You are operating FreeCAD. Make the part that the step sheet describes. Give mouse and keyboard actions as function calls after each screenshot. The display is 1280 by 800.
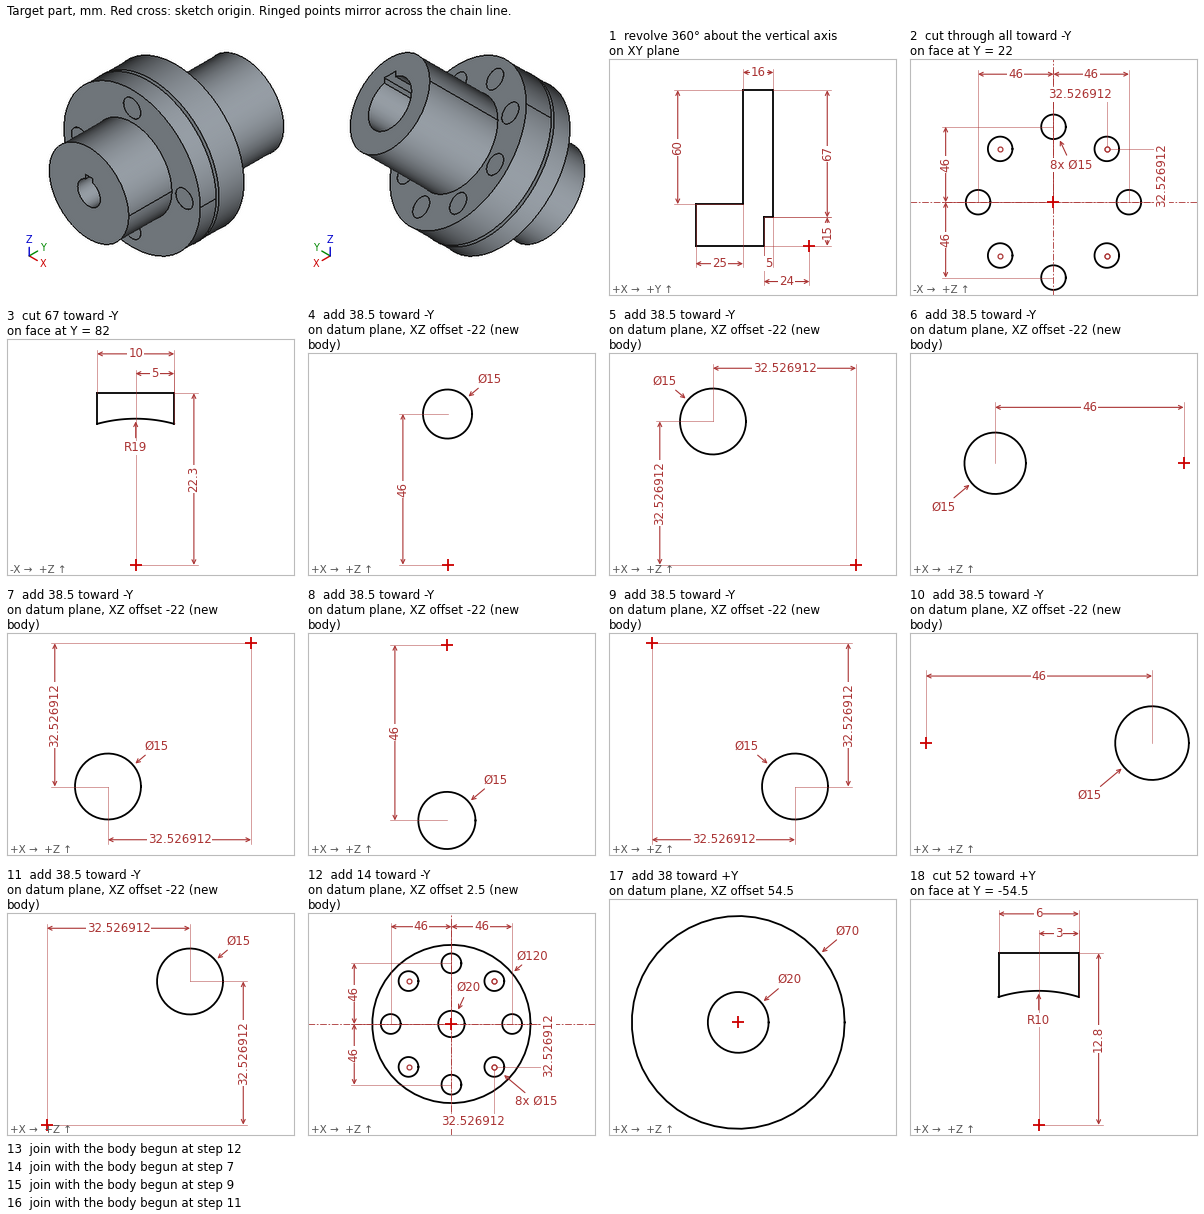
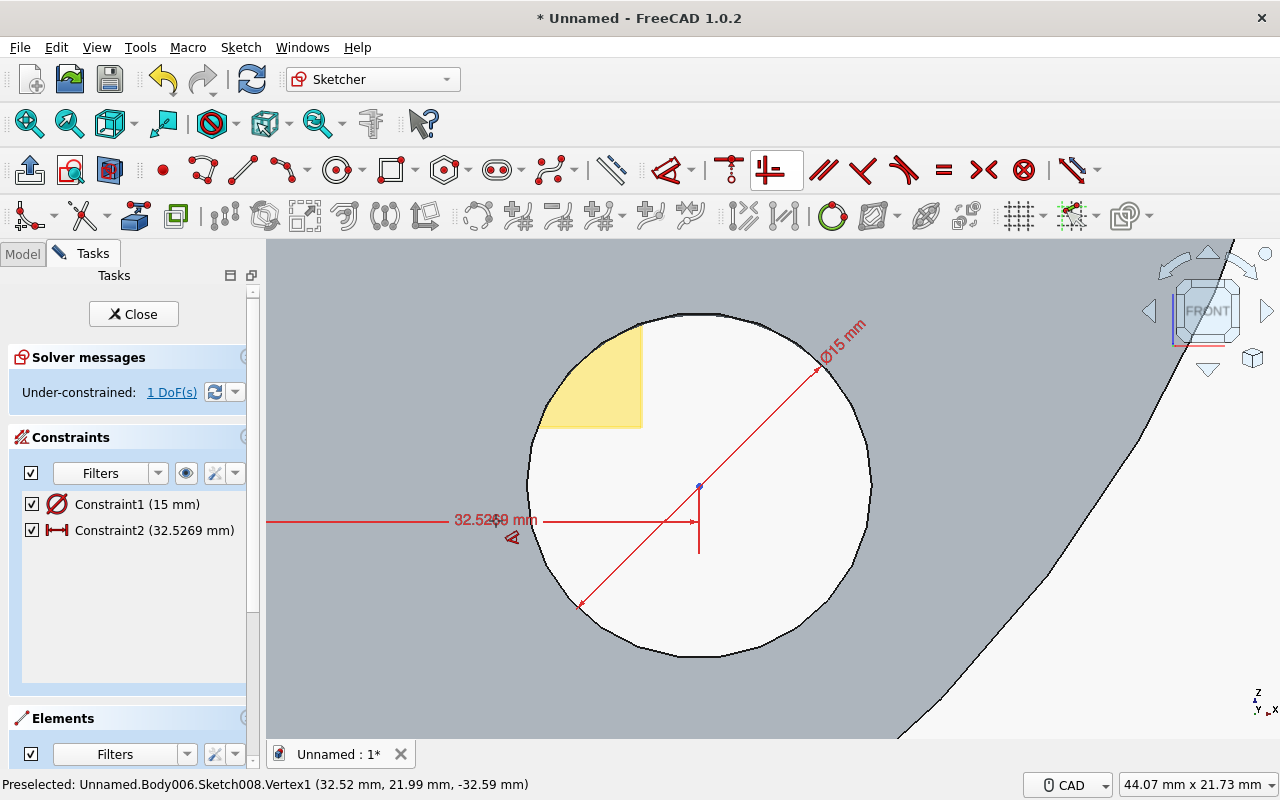
click(699, 487)
click(733, 377)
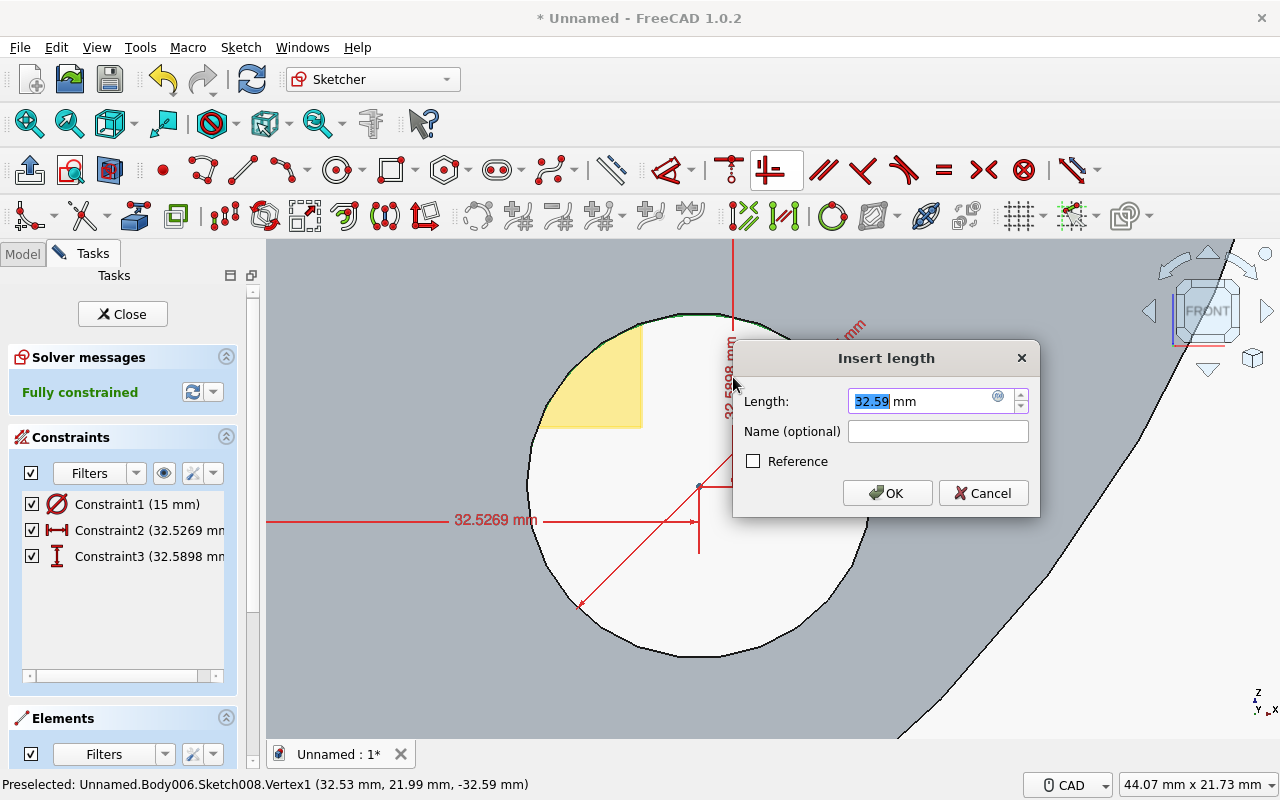
text(32.526912)
key(Return)
key(Escape)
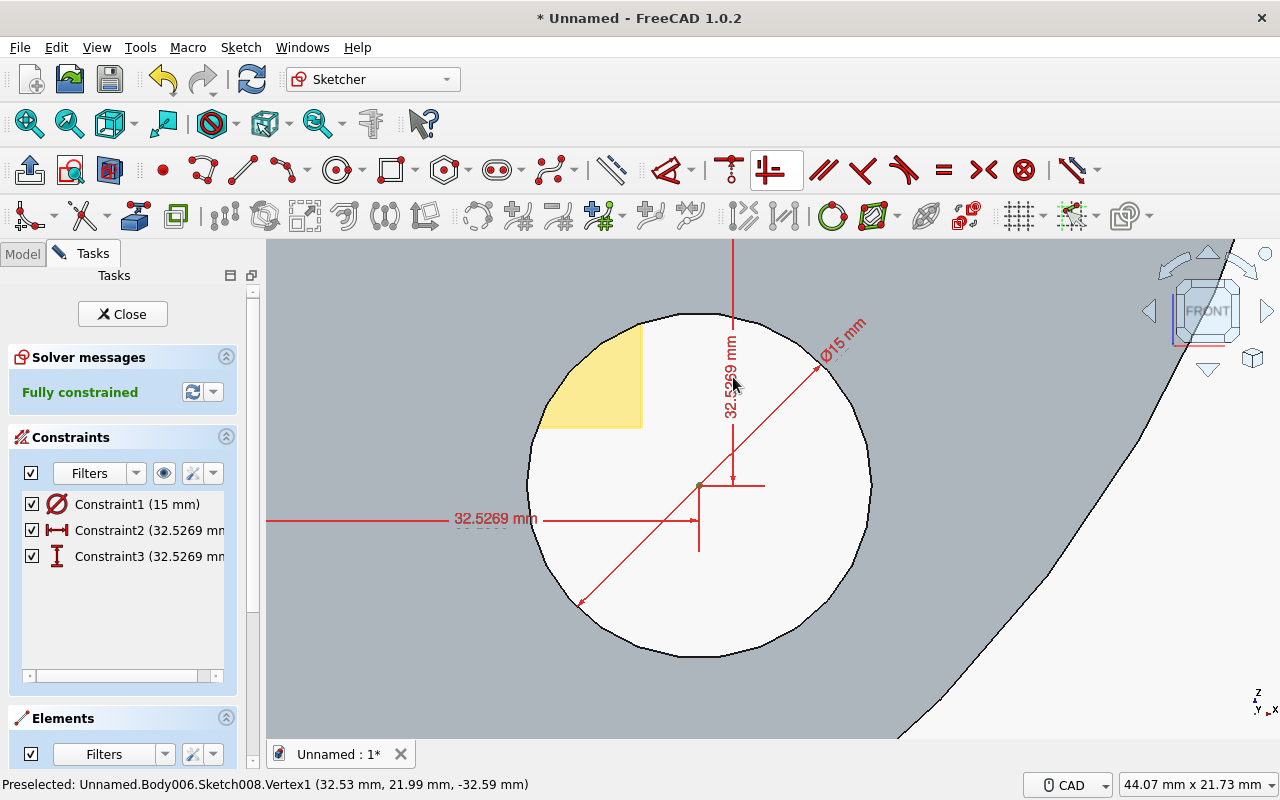
click(123, 314)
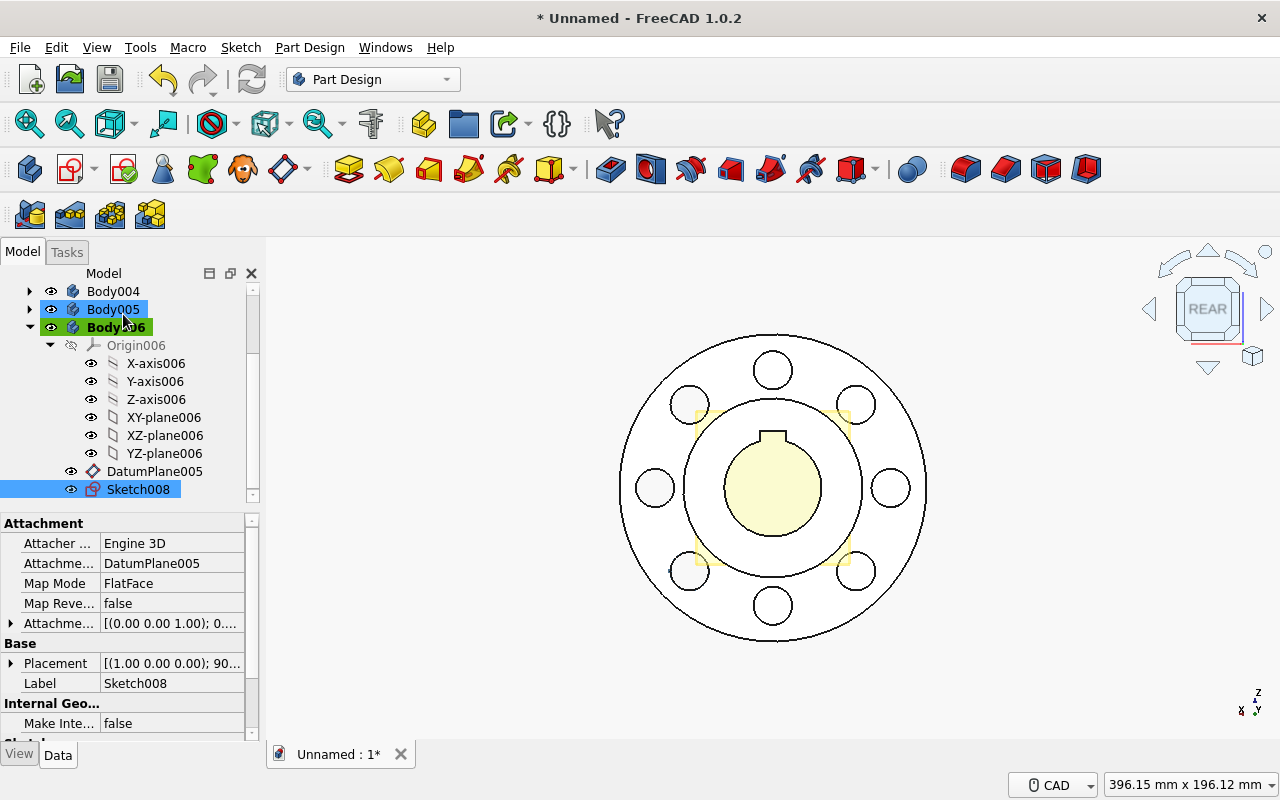
click(350, 170)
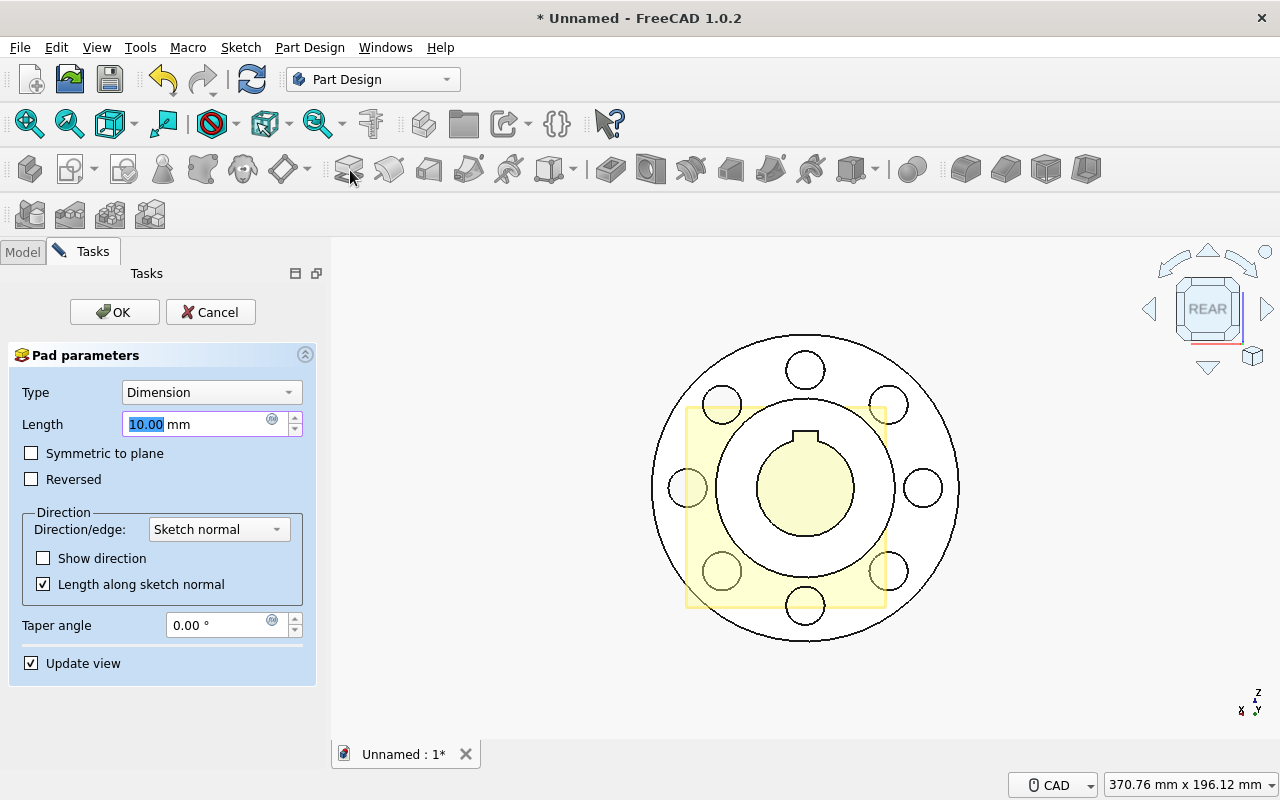
text(38.5)
key(Tab)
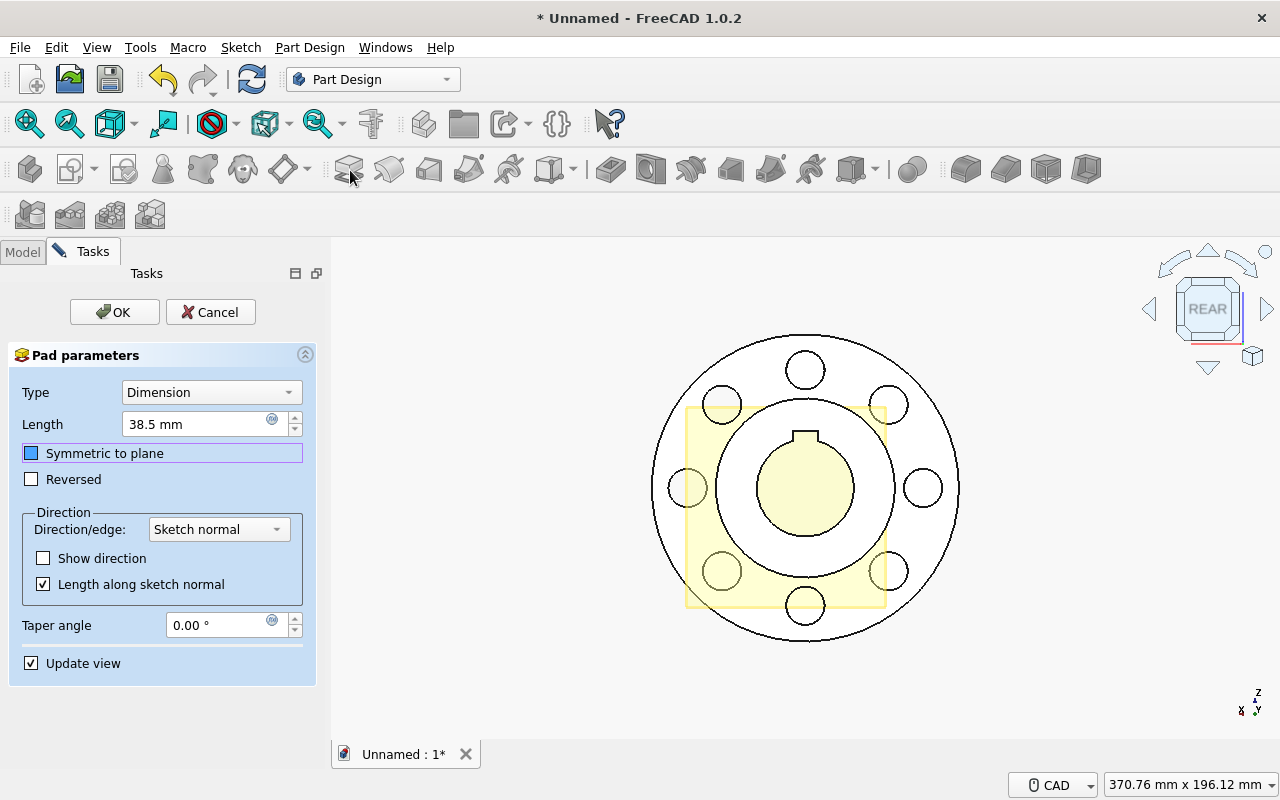
click(115, 312)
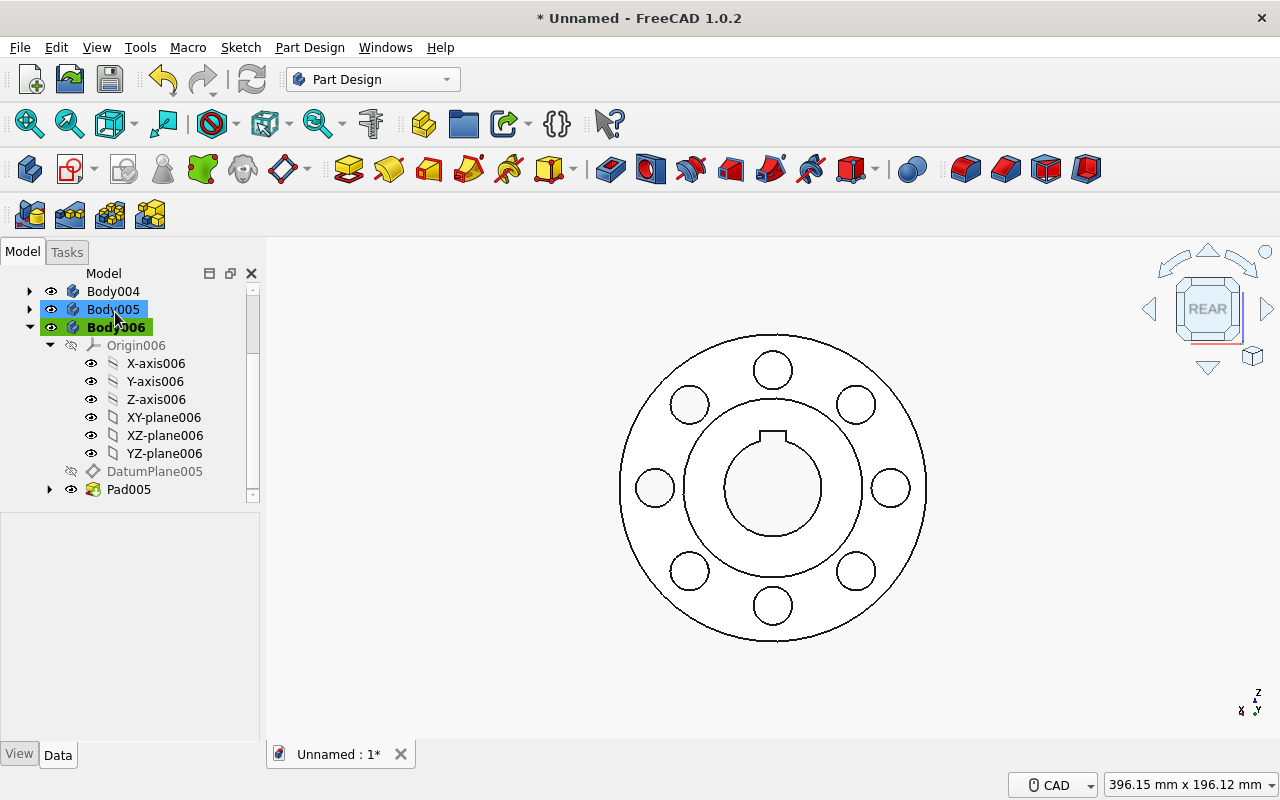
click(30, 124)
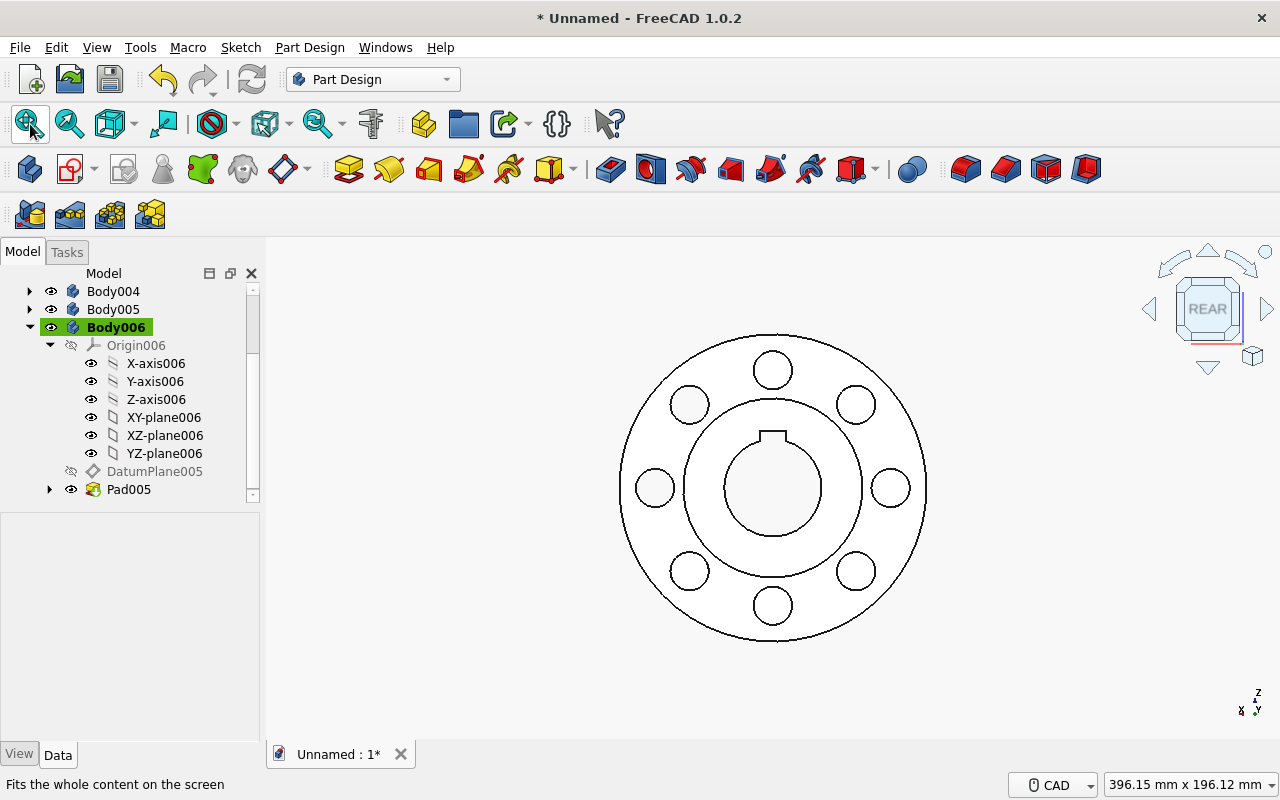
click(30, 170)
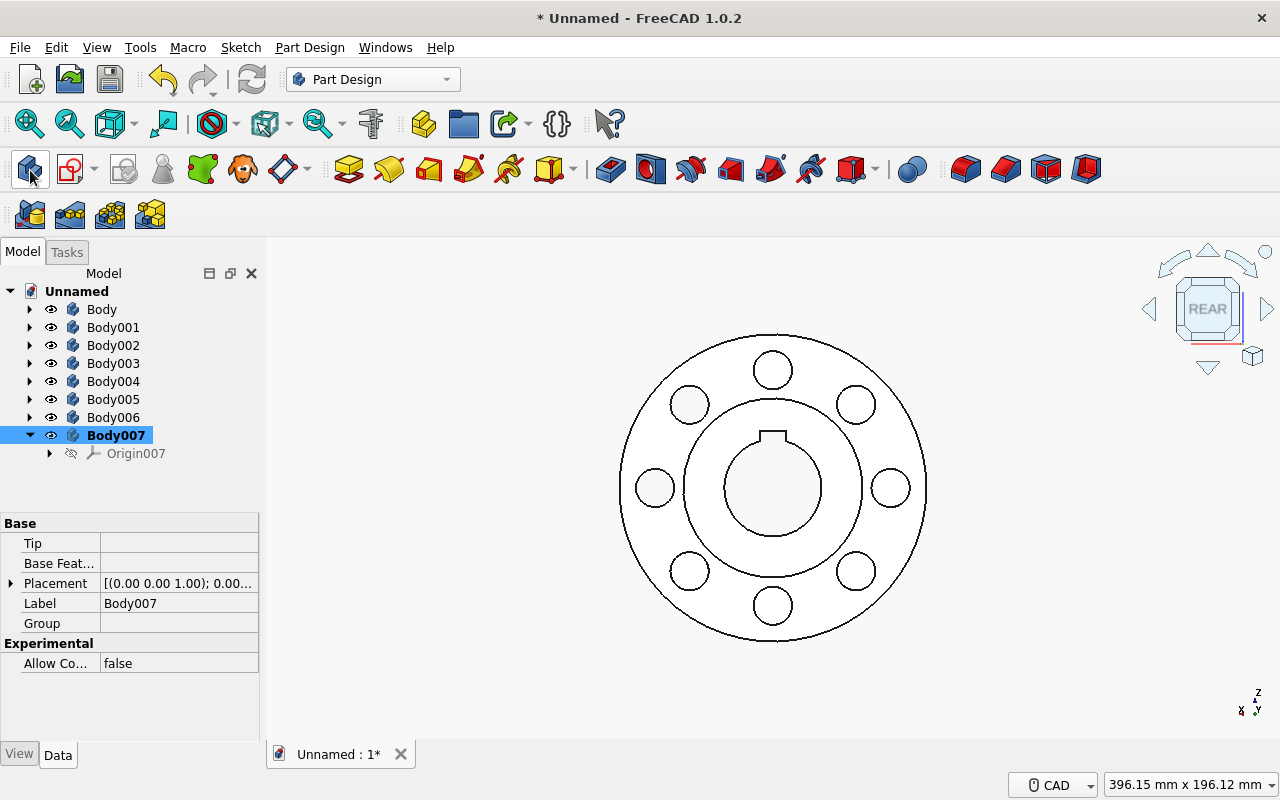
click(50, 453)